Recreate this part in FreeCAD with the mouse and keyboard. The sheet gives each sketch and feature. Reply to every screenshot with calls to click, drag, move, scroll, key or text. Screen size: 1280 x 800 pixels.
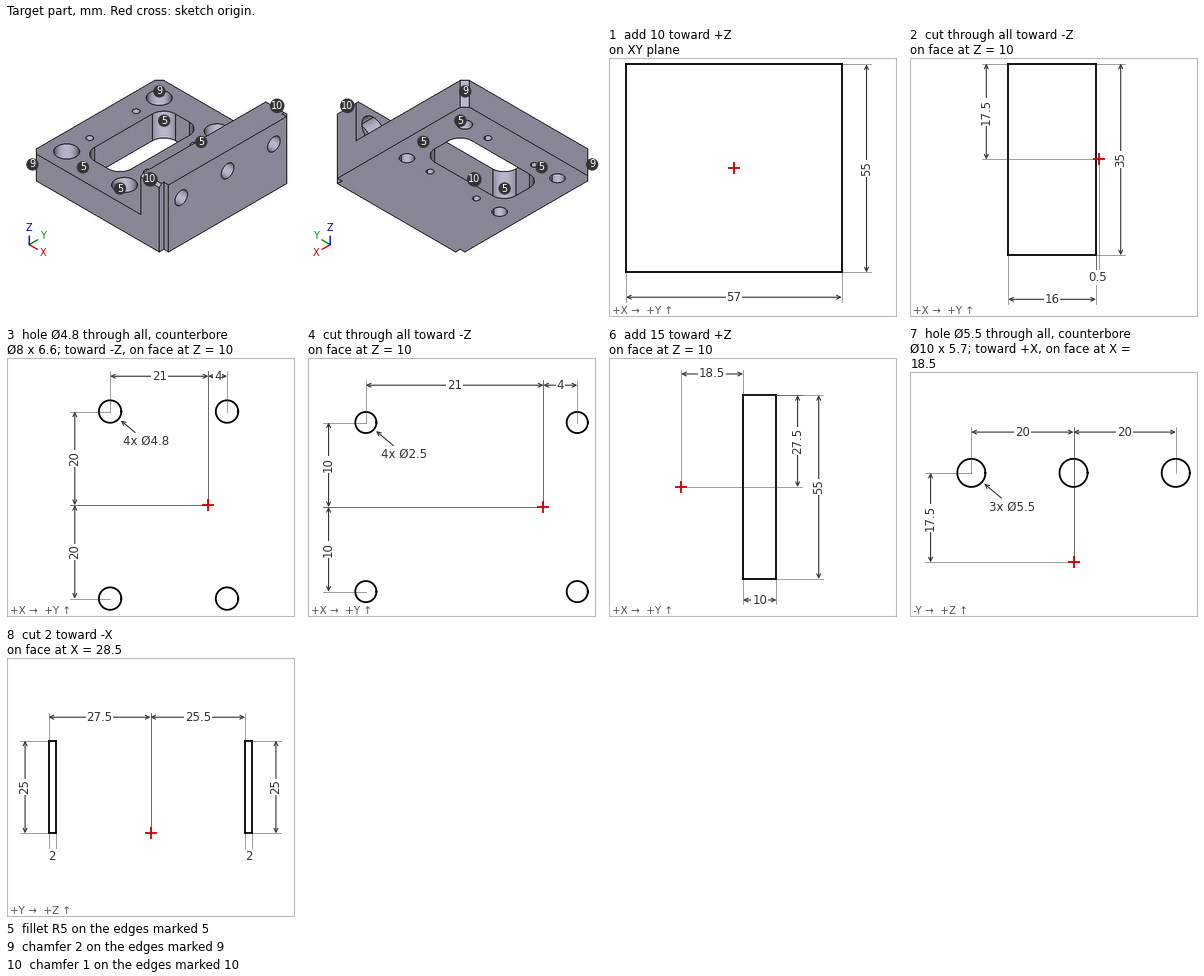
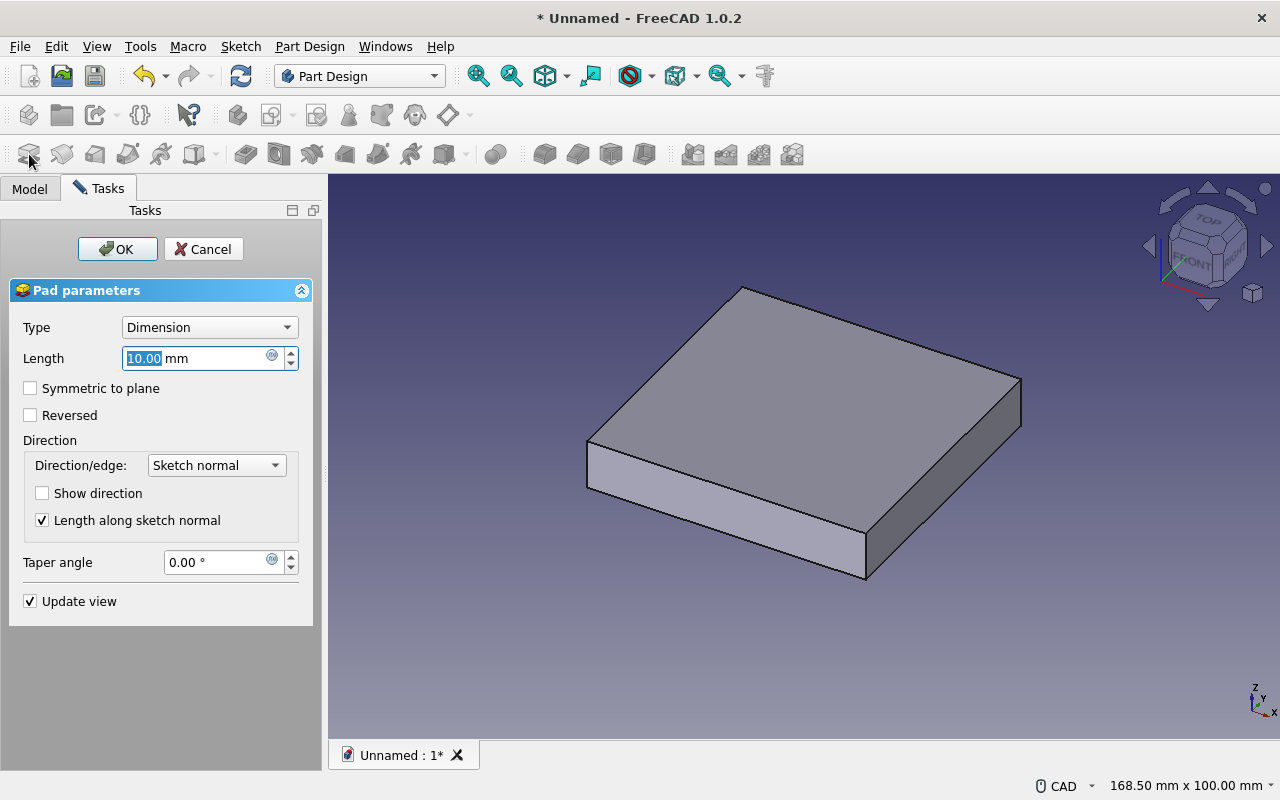
text(10)
key(Tab)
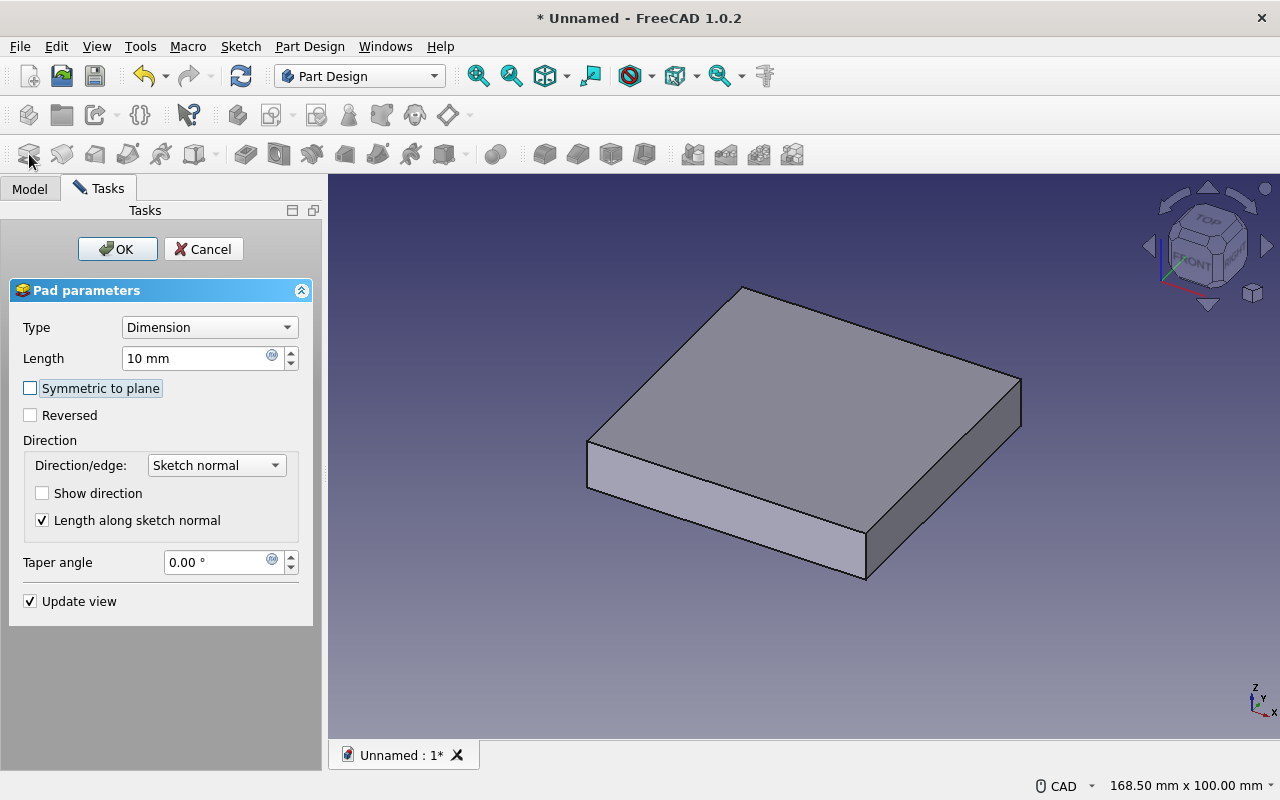
click(118, 249)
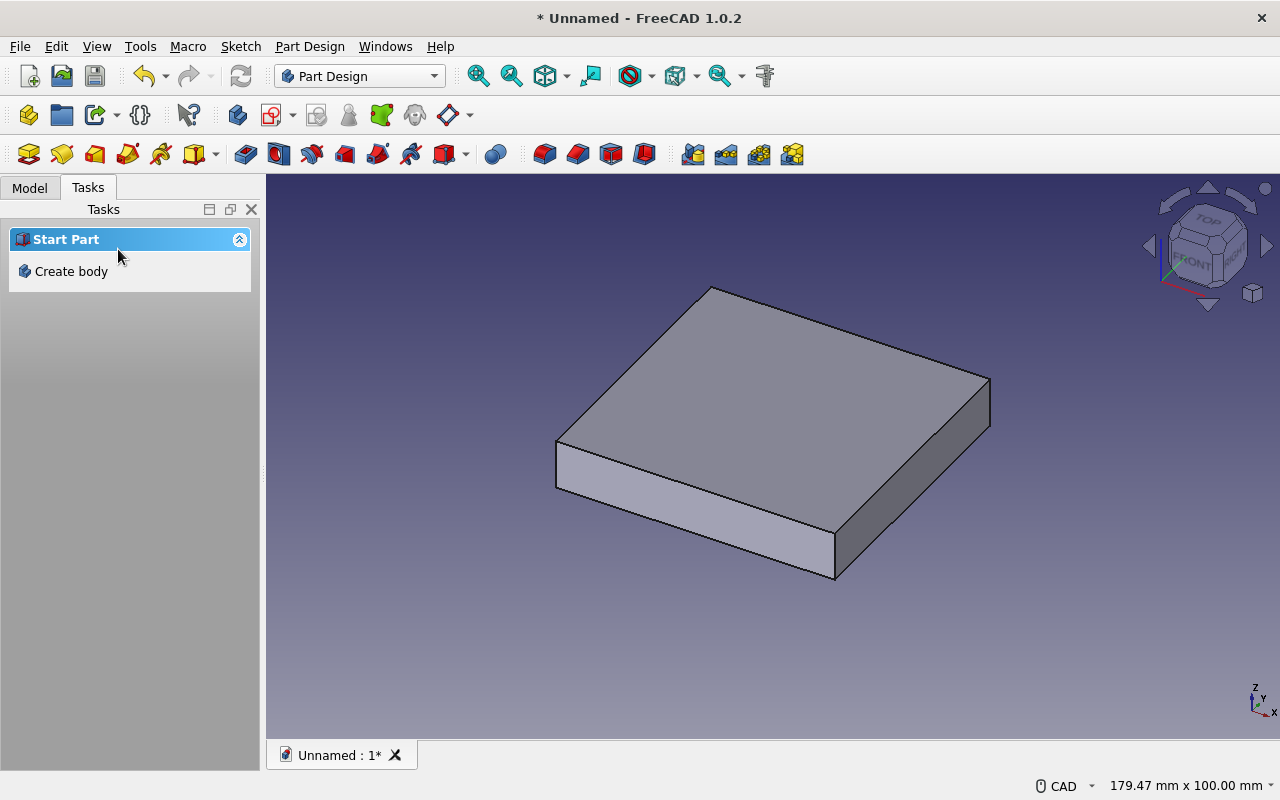
click(773, 409)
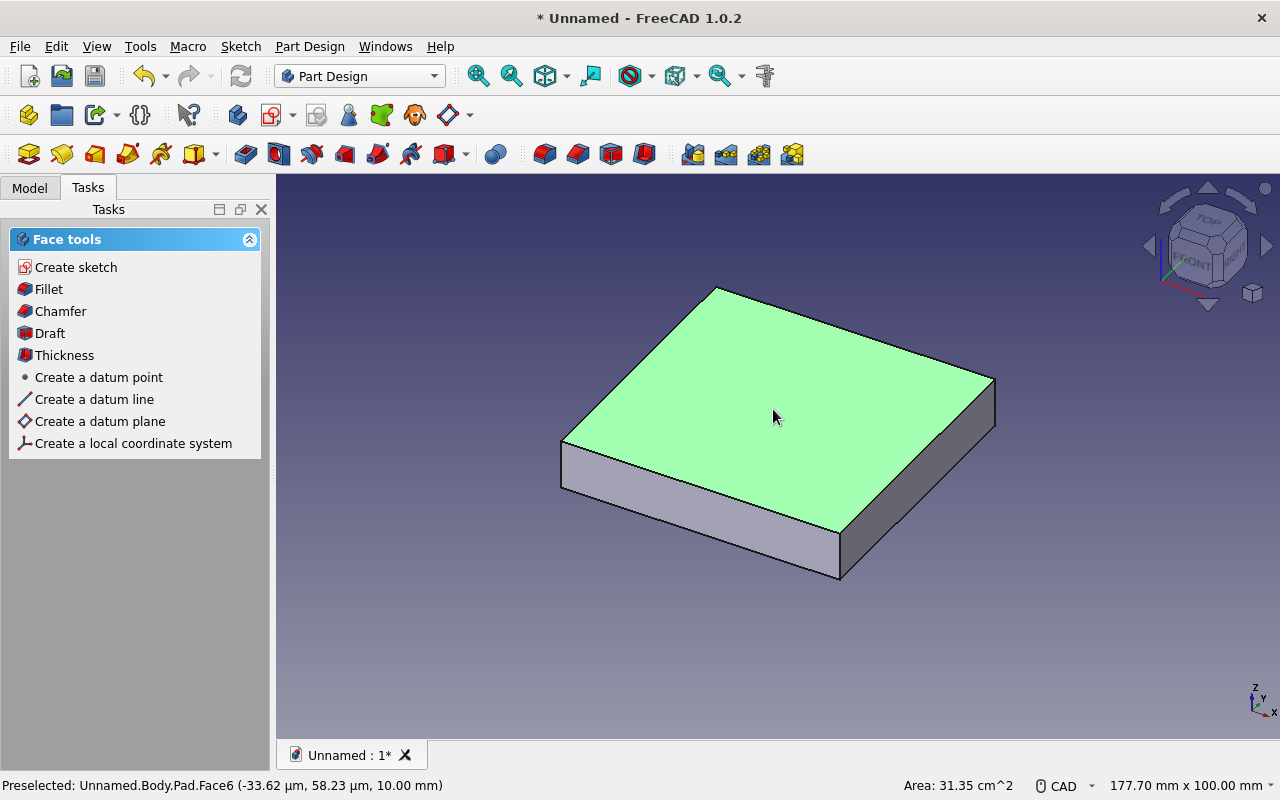
click(270, 116)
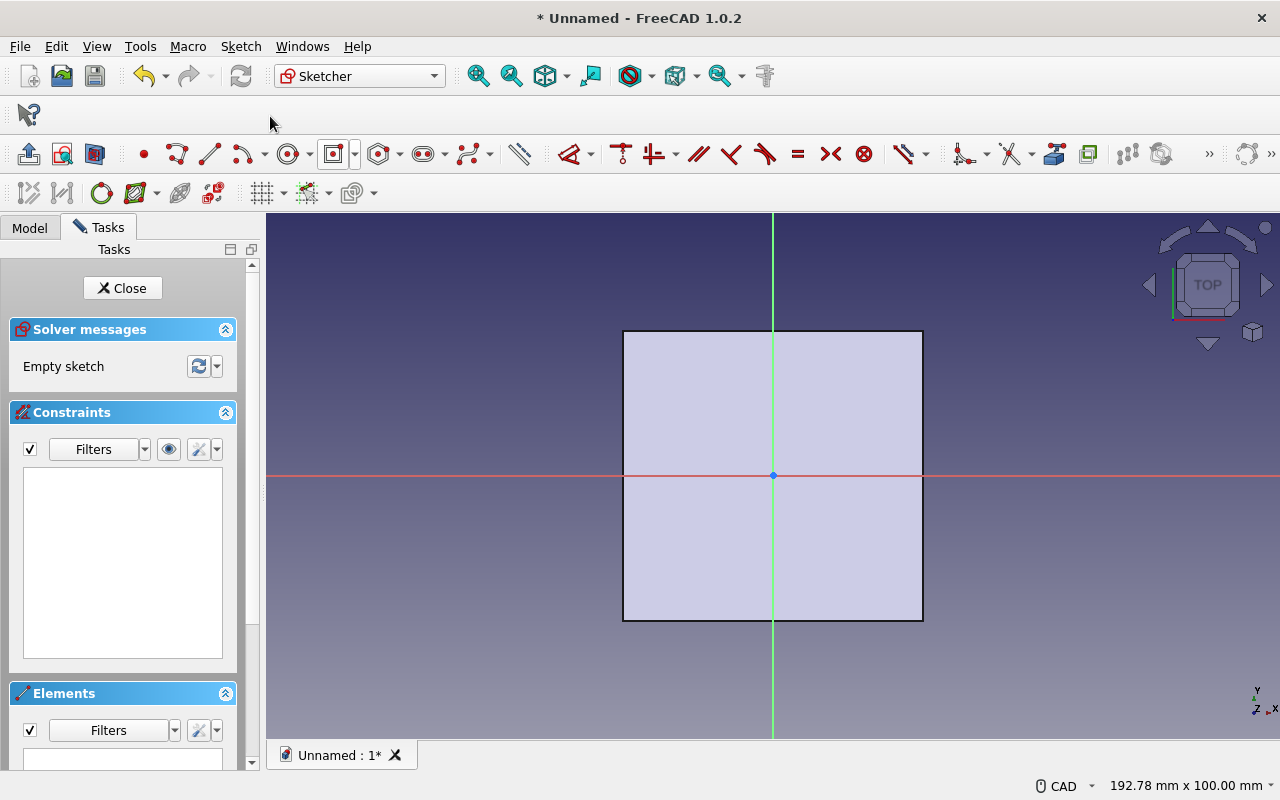
scroll(760, 476, up, 3)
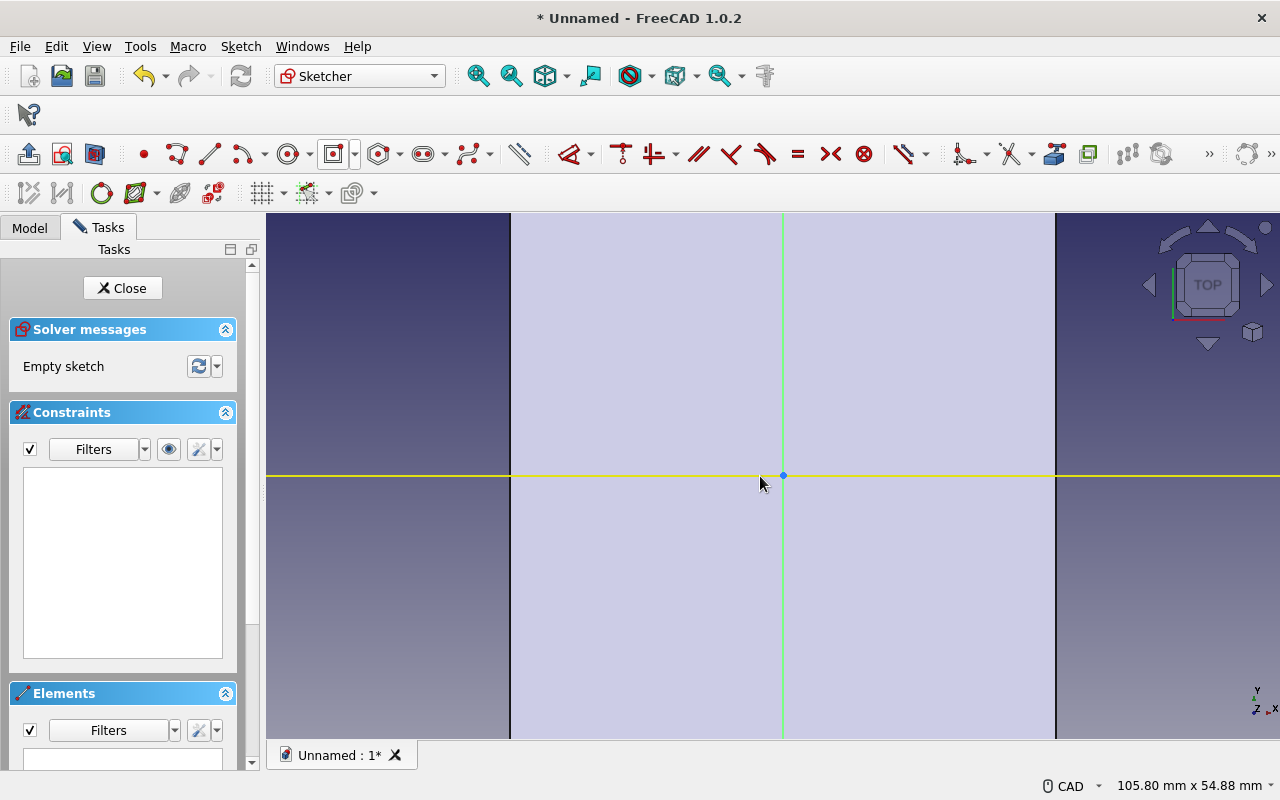
click(354, 154)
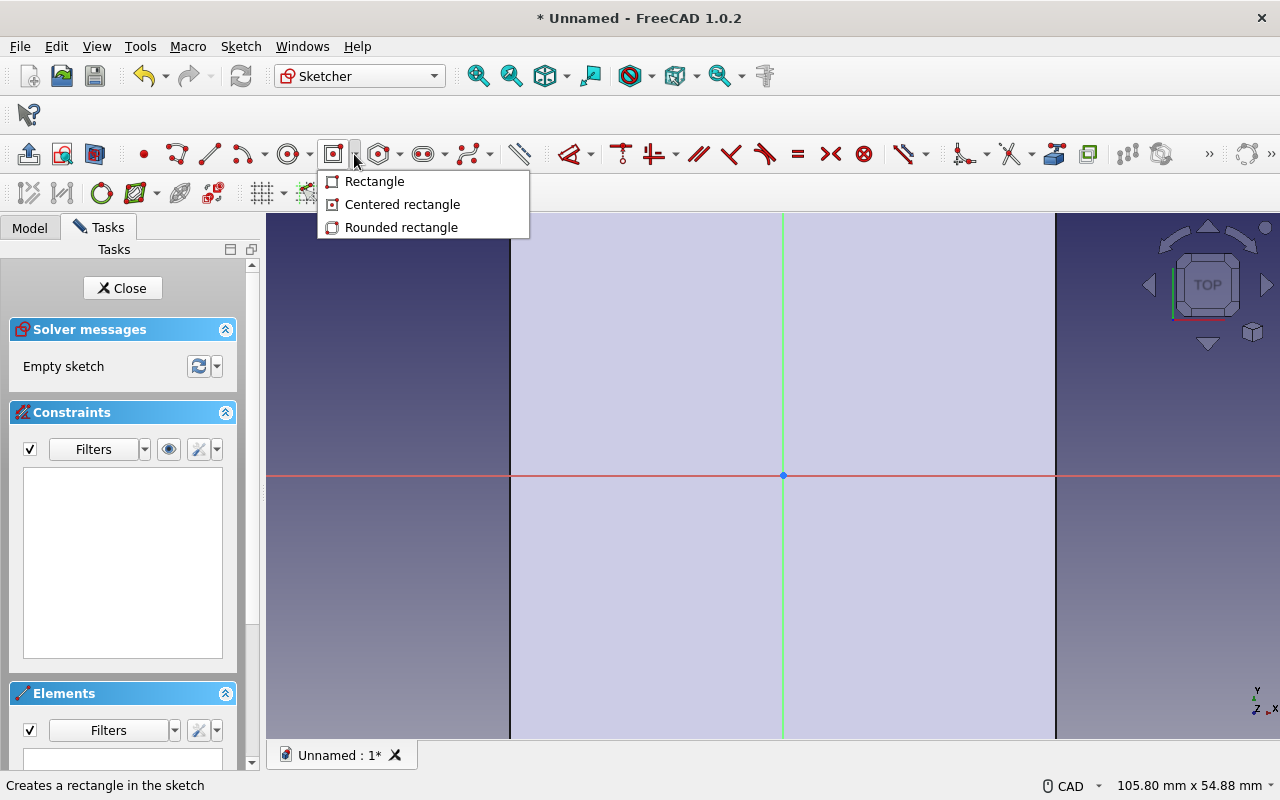
click(424, 182)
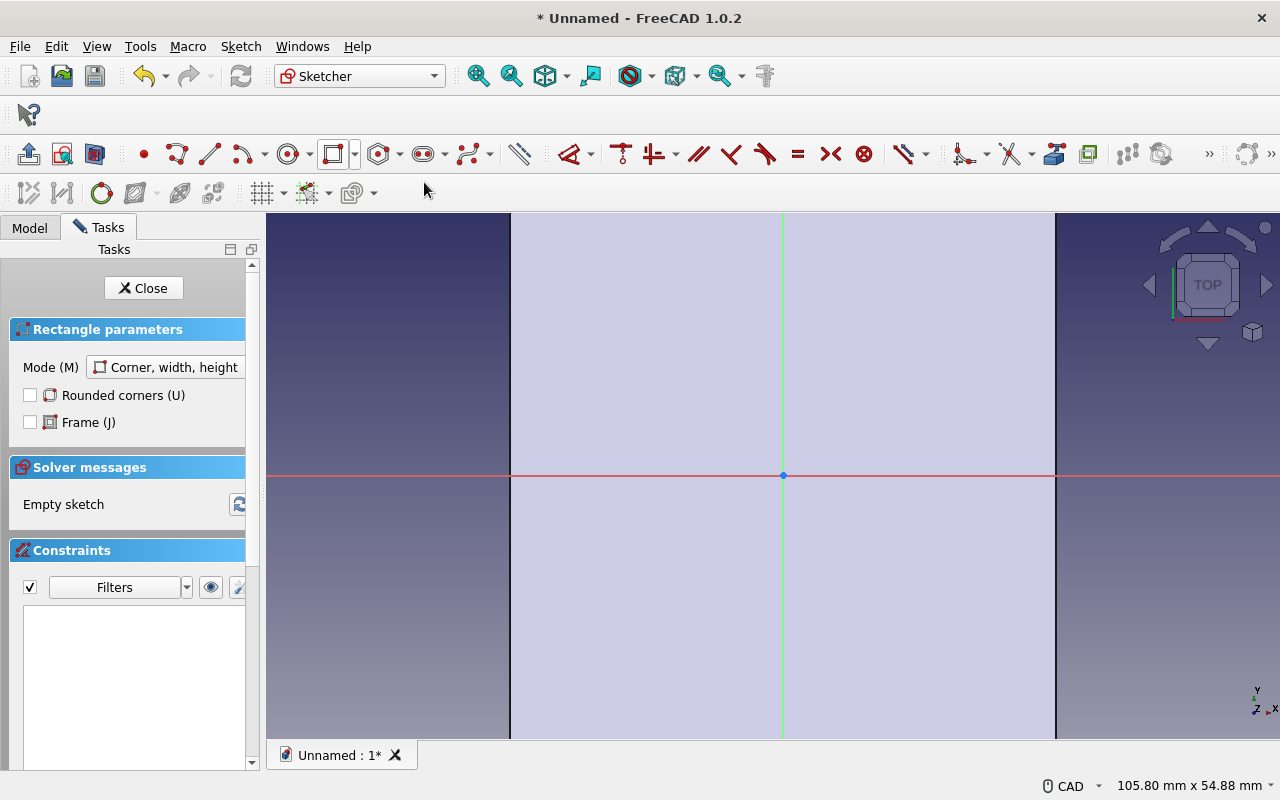
click(625, 308)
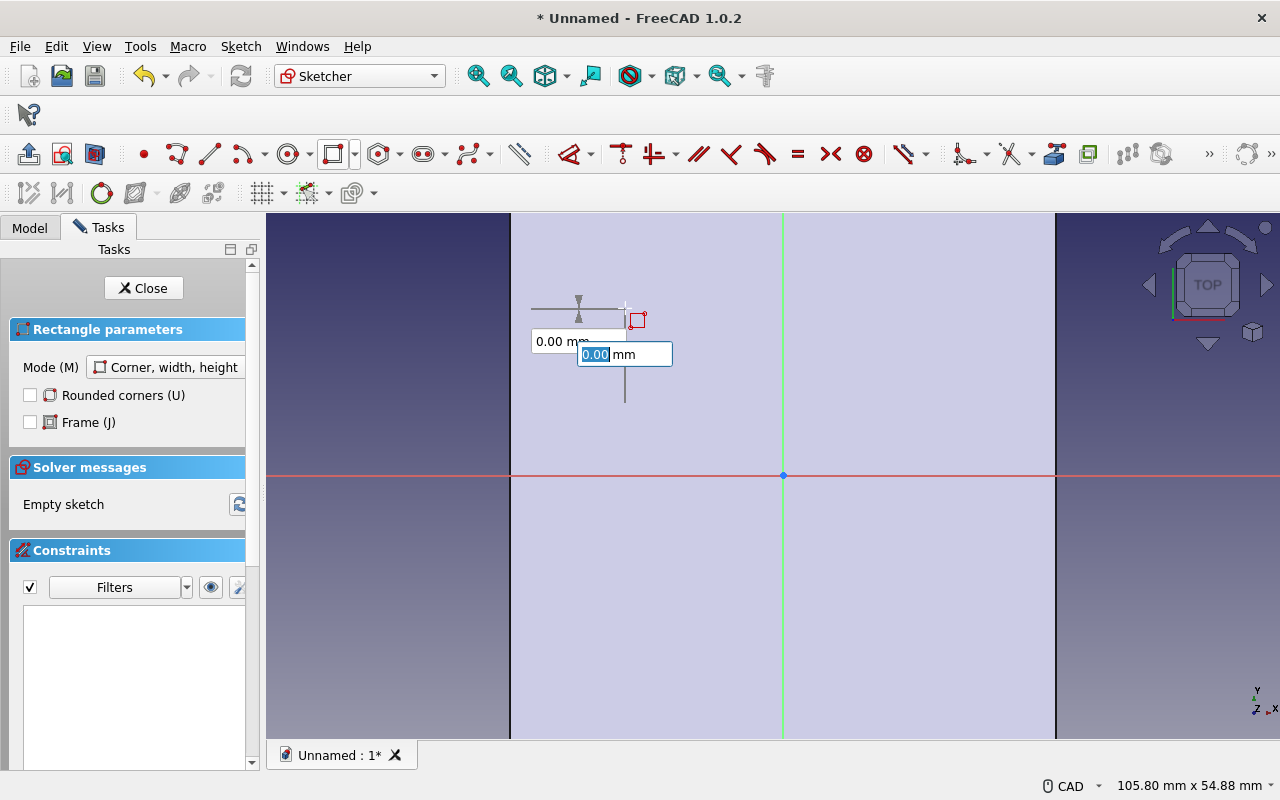
scroll(778, 643, up, 6)
move(778, 642)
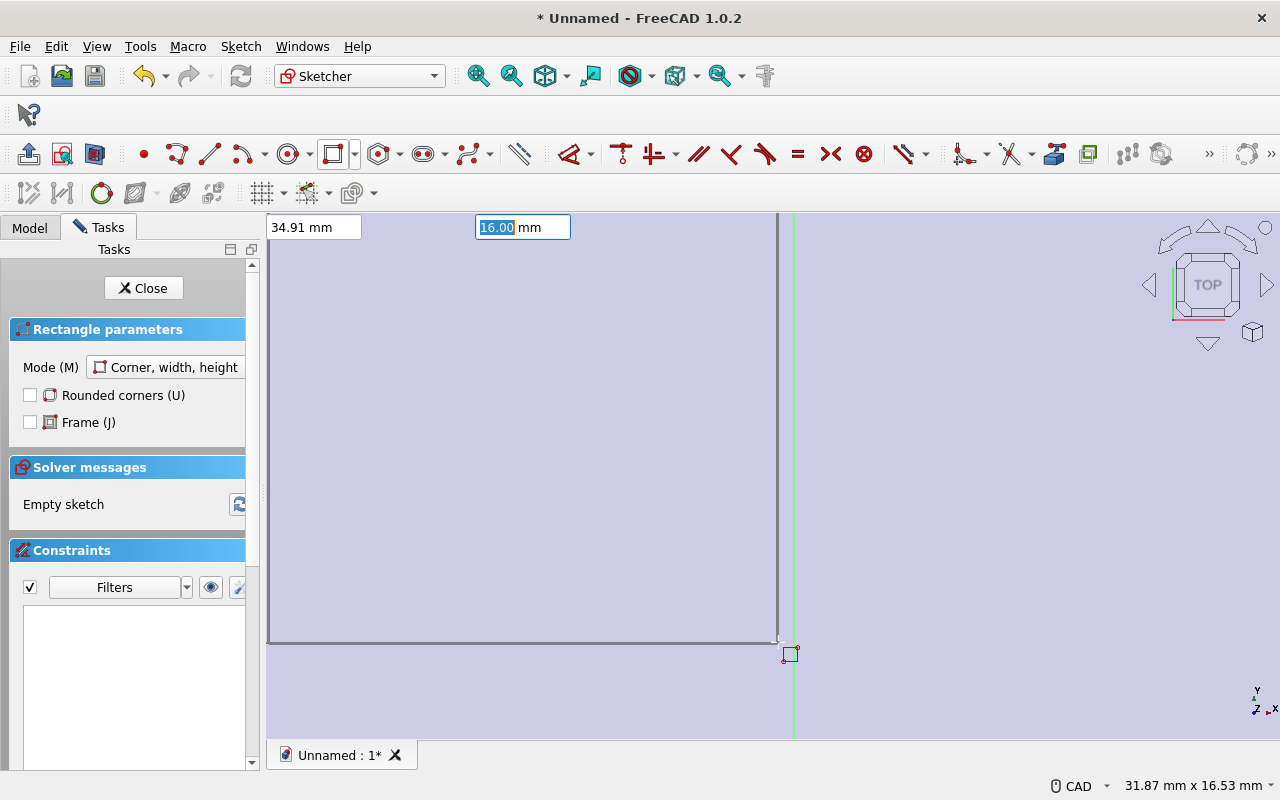
text(16)
key(Tab)
text(35)
key(Return)
key(Escape)